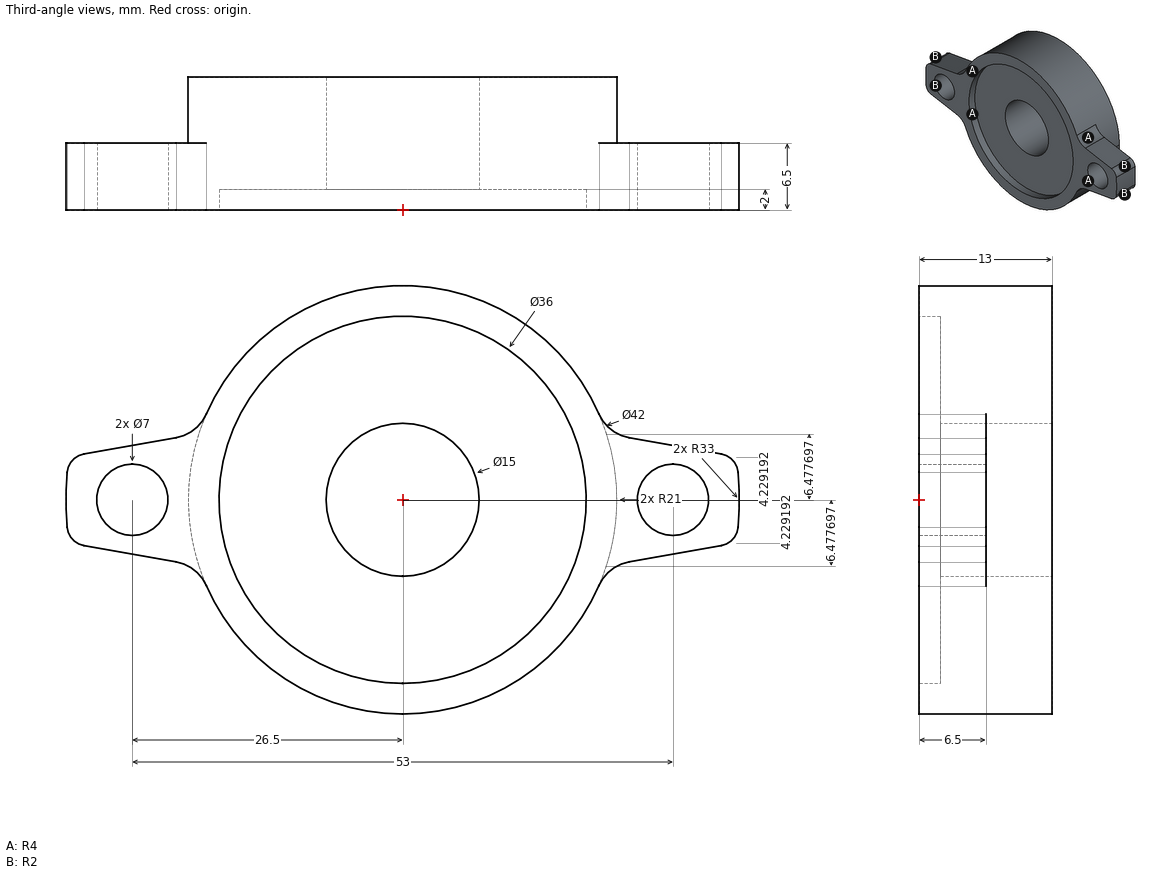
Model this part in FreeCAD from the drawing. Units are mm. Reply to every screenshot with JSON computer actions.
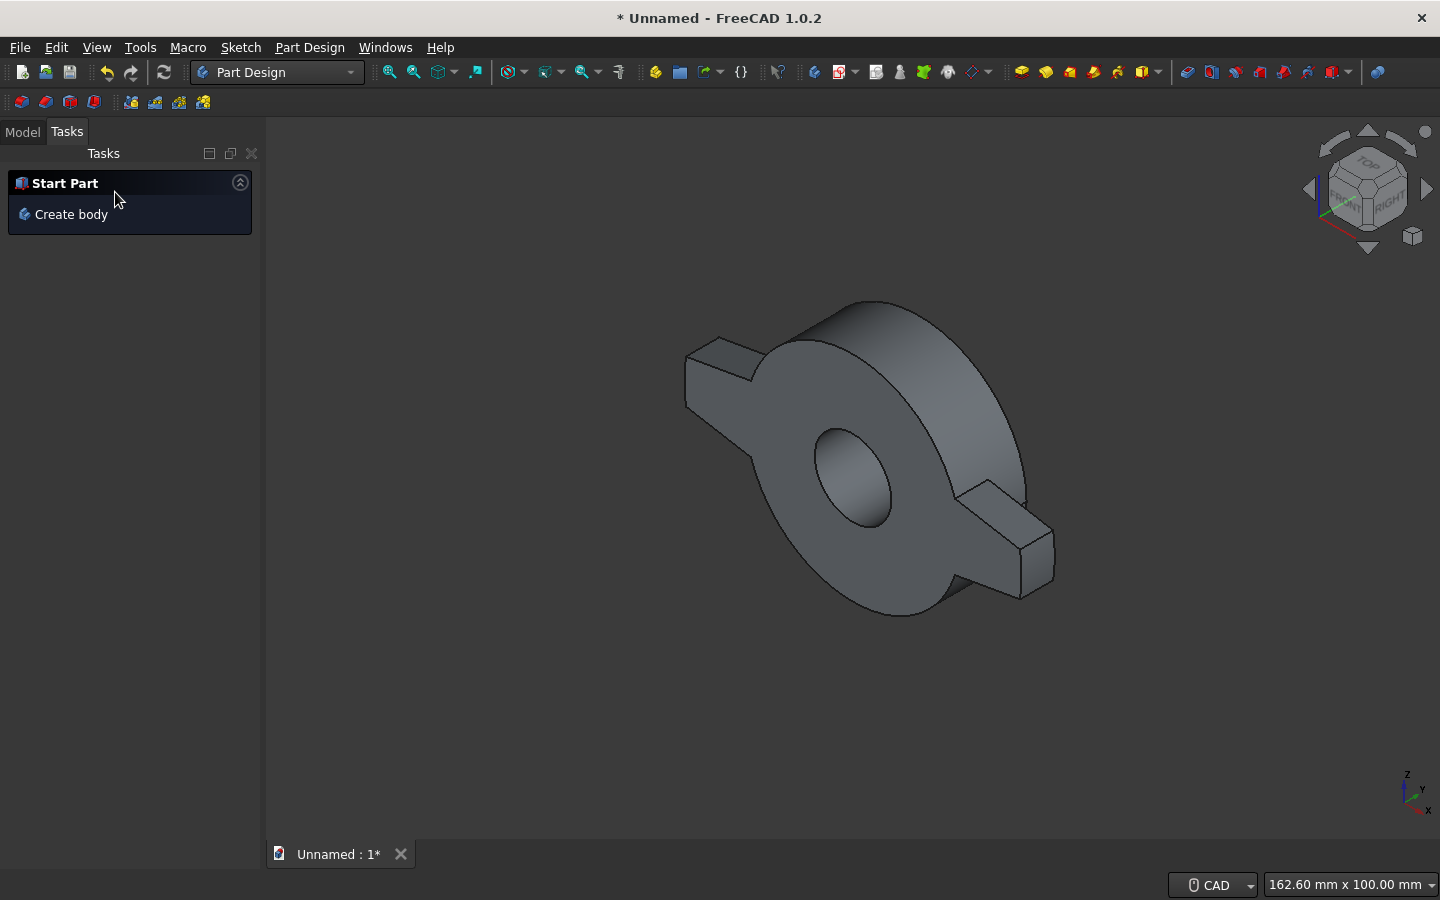
{"action": "key", "text": "2"}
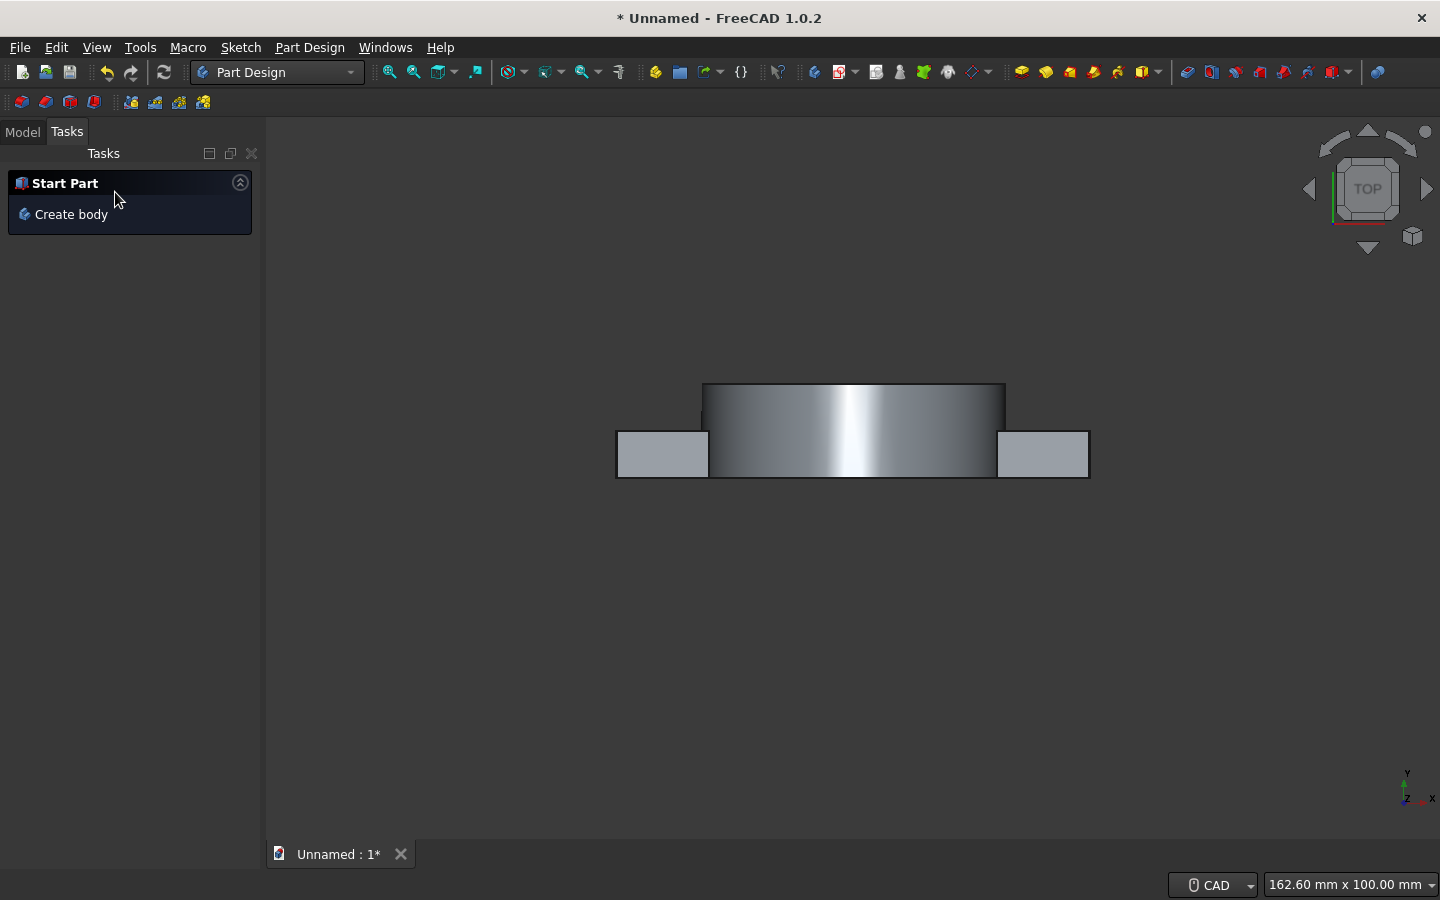
{"action": "left_click", "coordinate": [390, 72]}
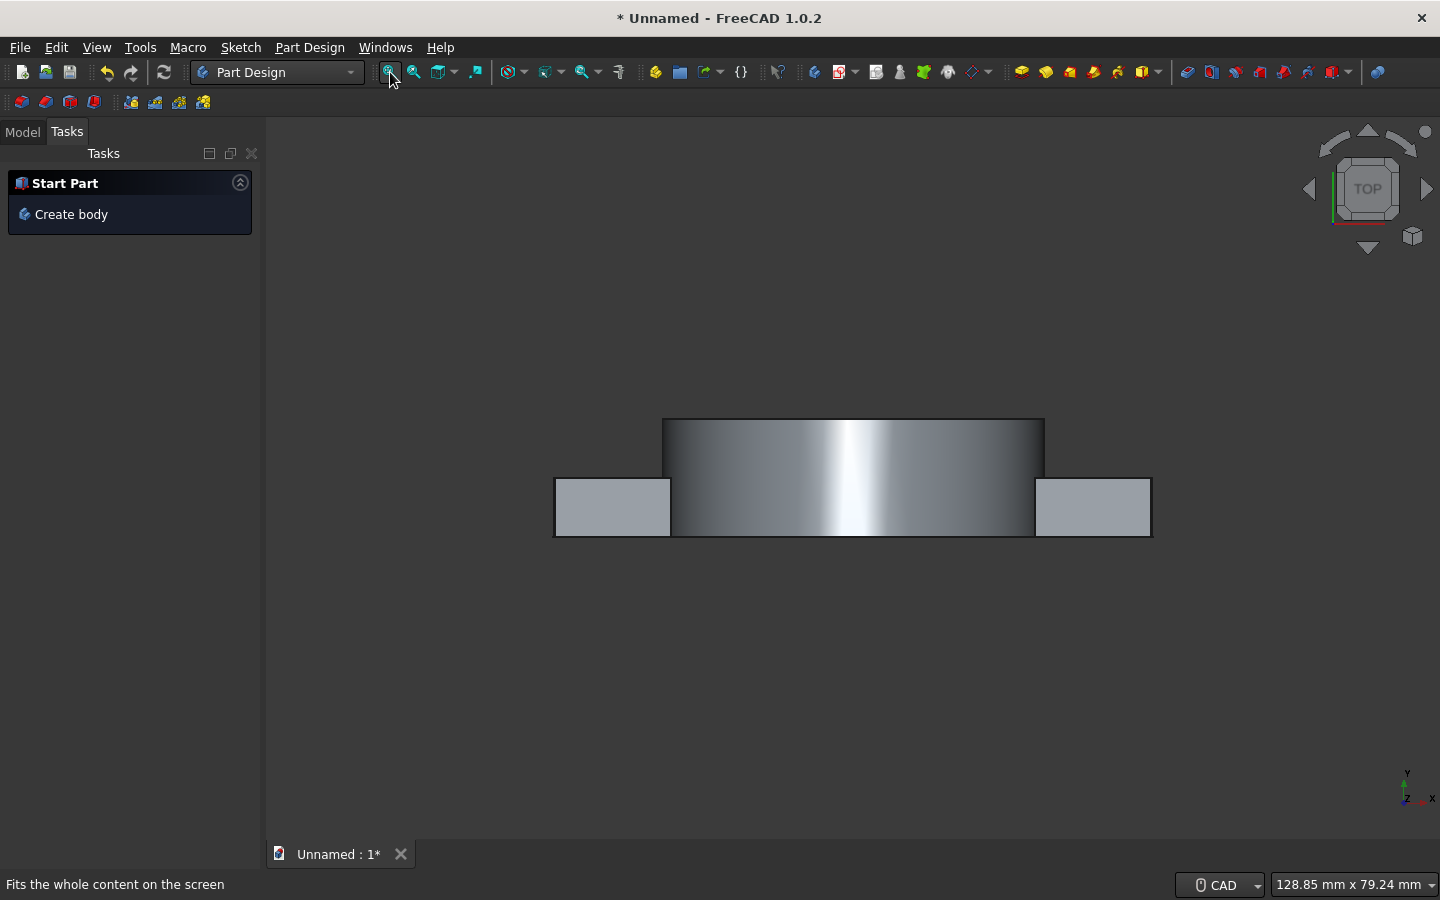
{"action": "key", "text": "1"}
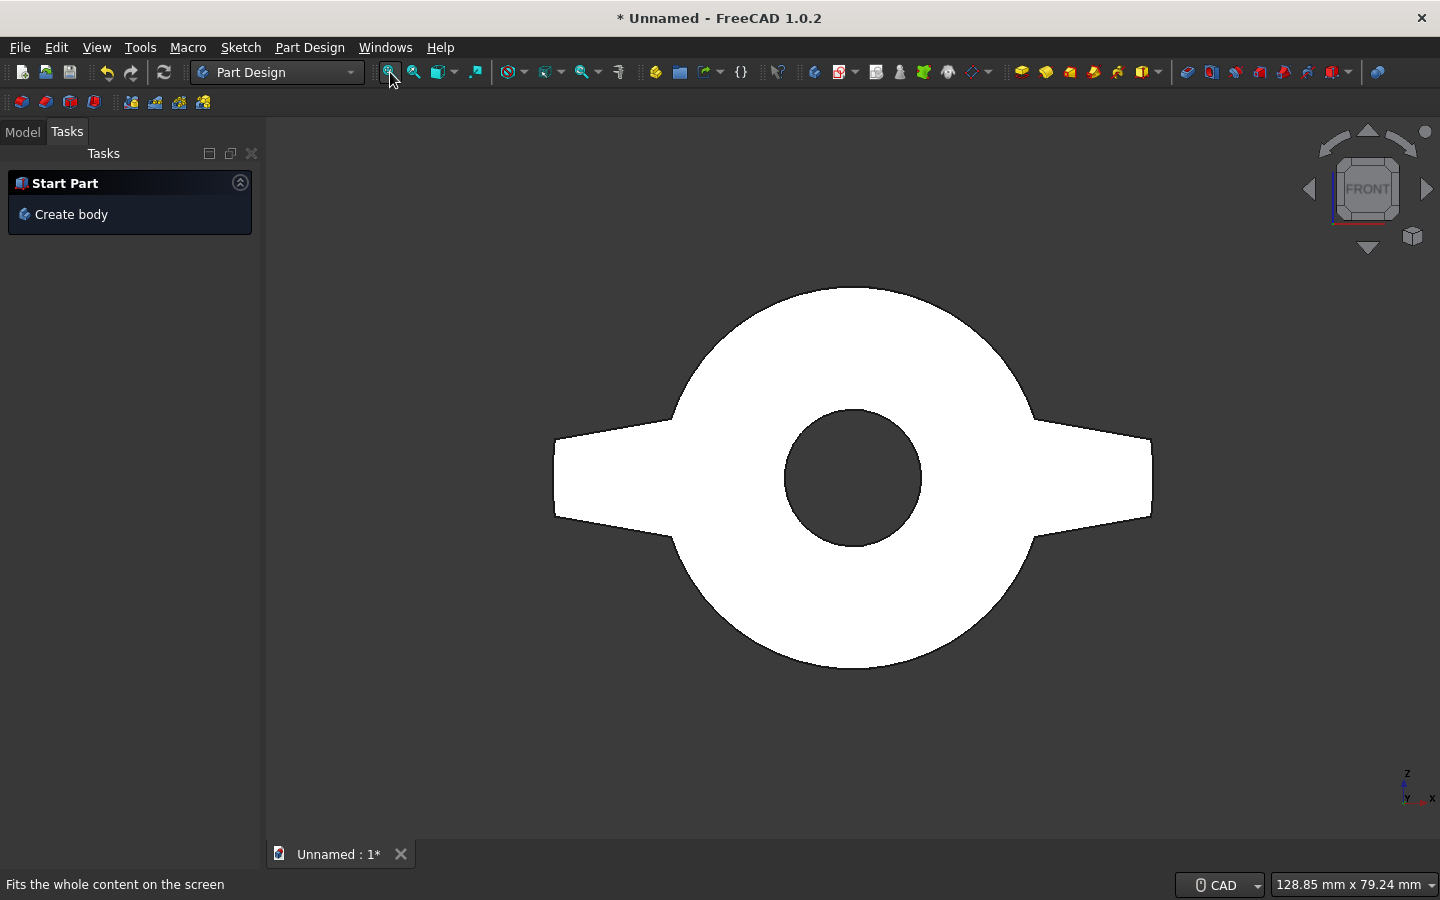
{"action": "key", "text": "3"}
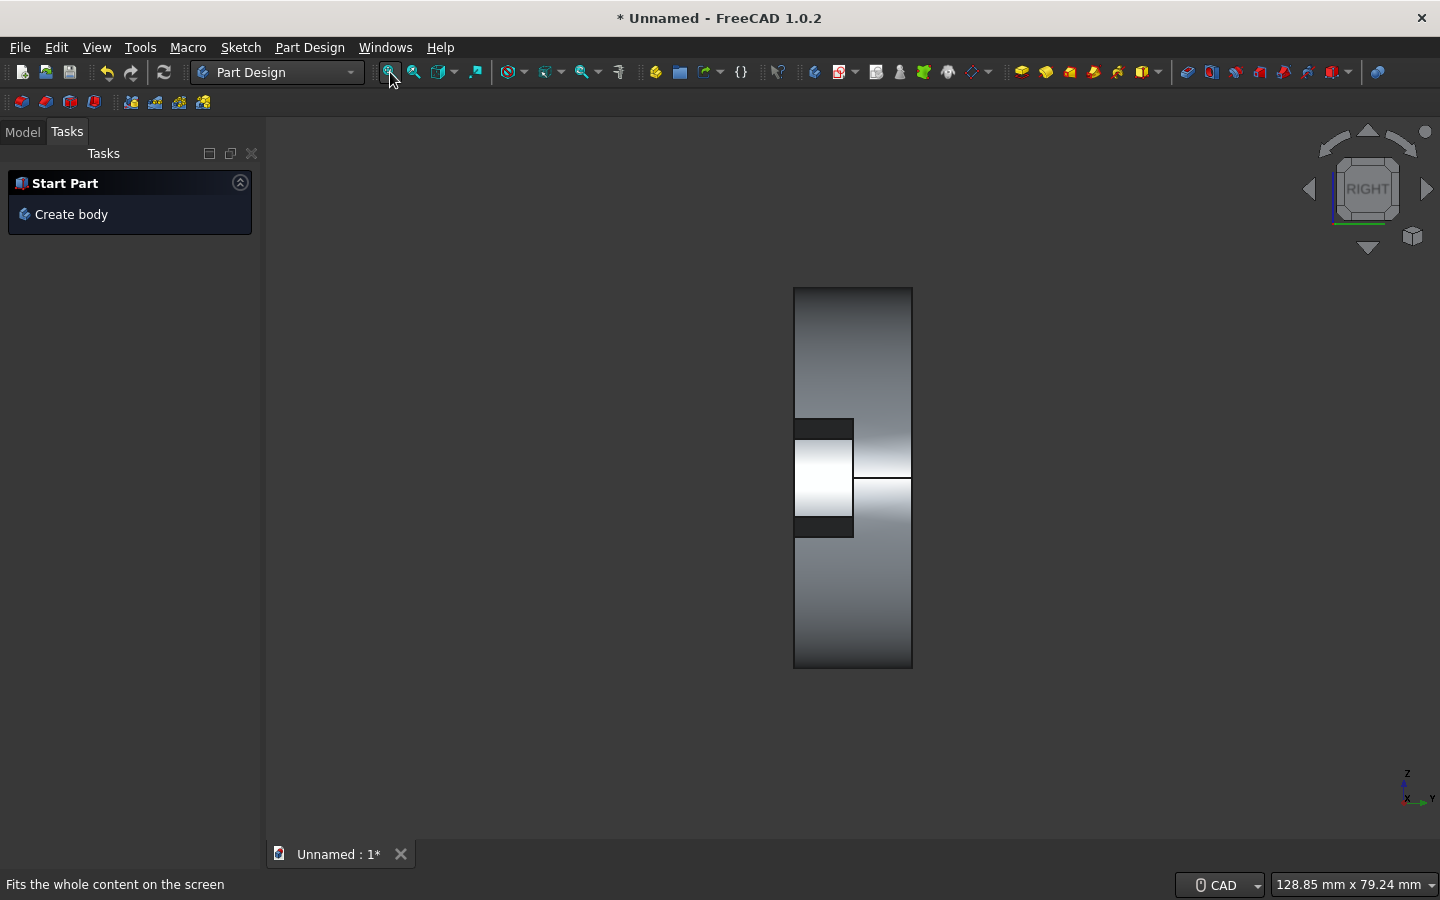
{"action": "key", "text": "5"}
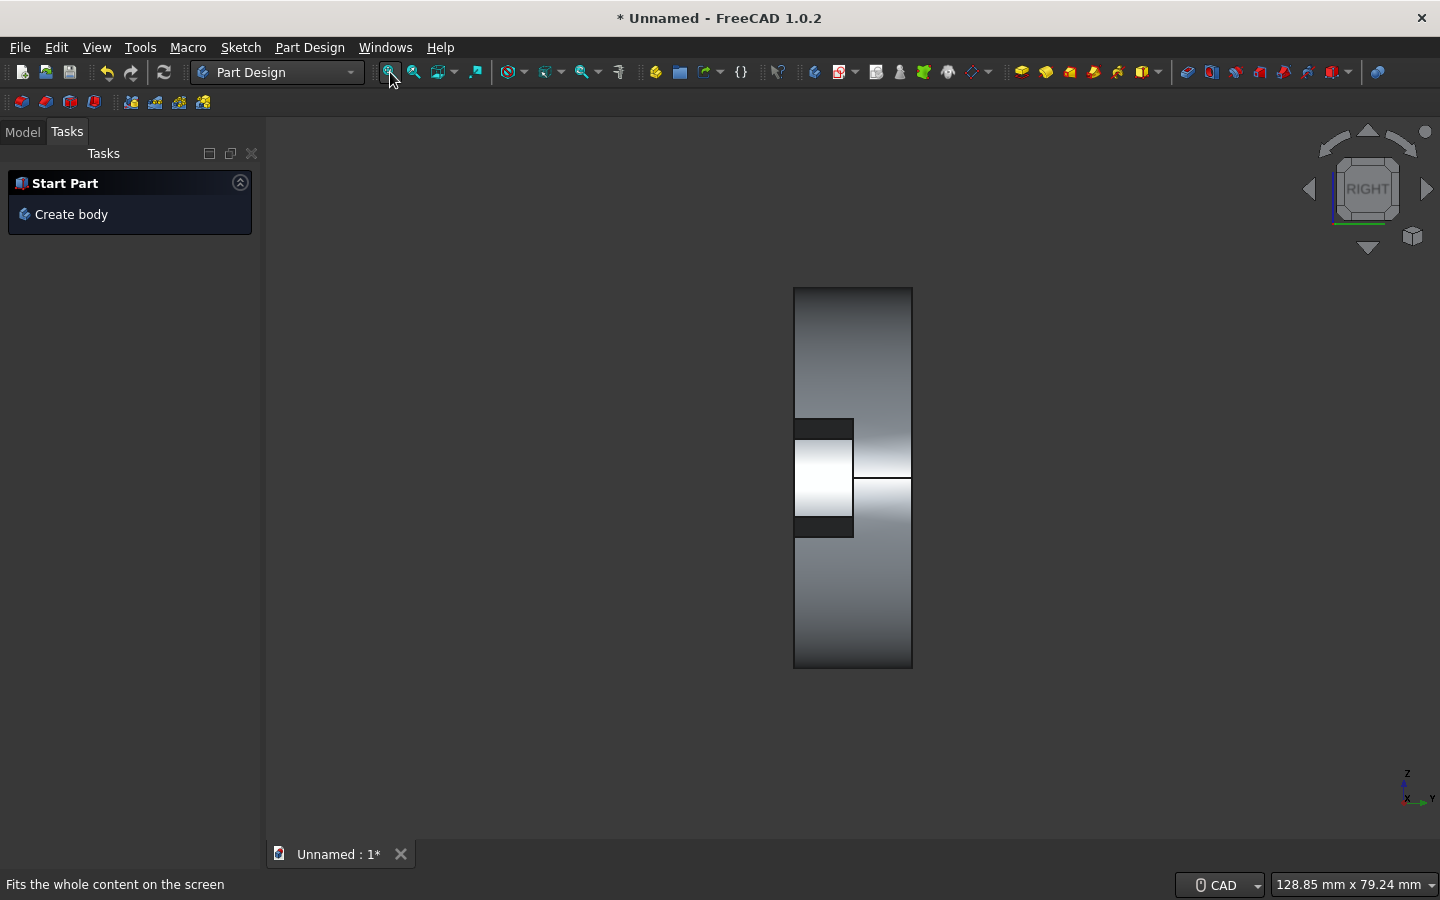
{"action": "key", "text": "4"}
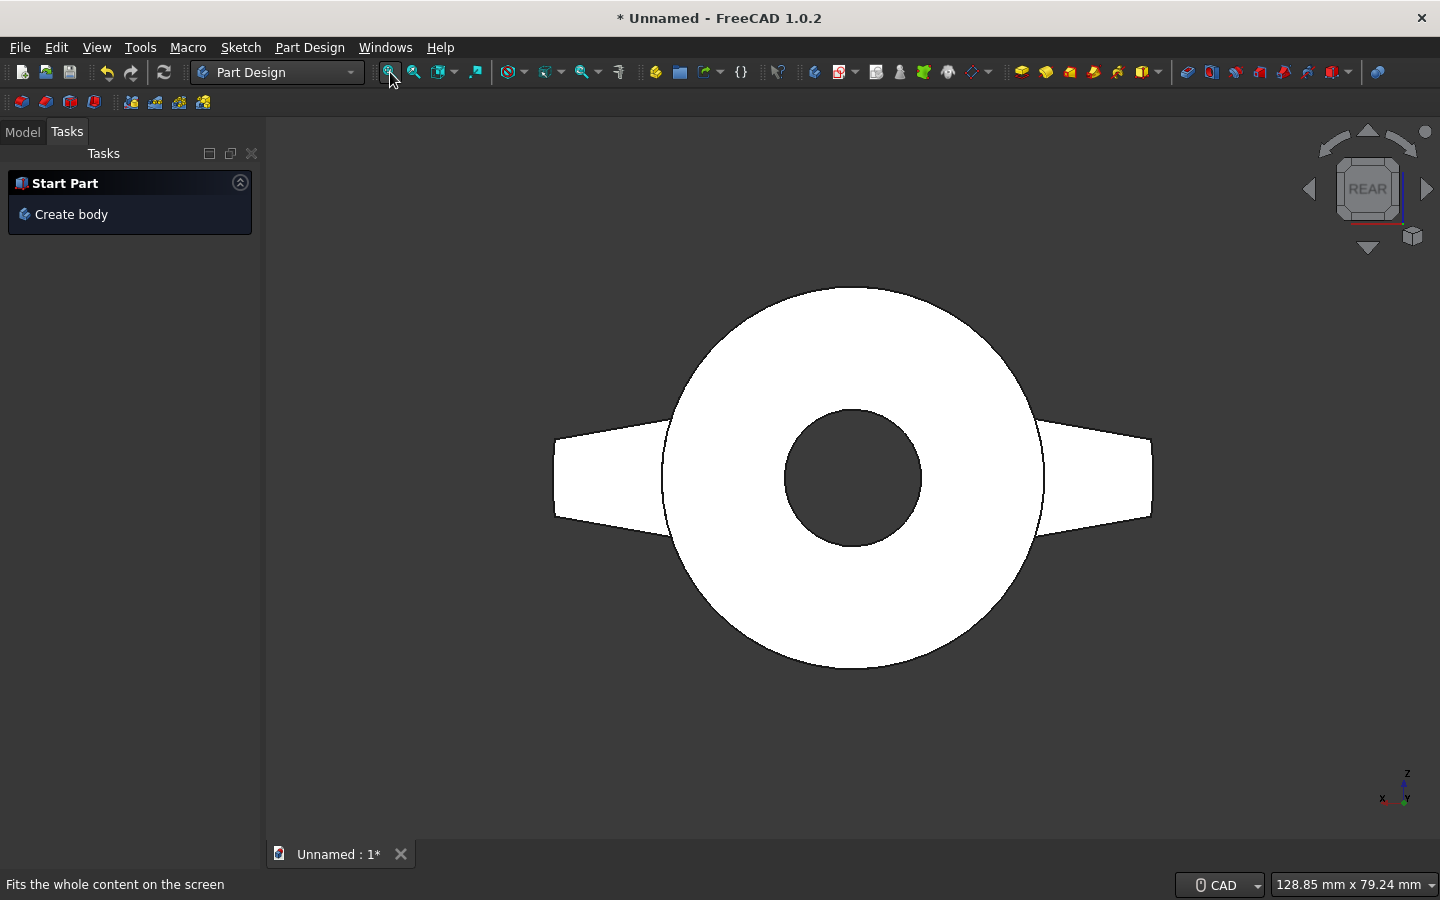
{"action": "key", "text": "6"}